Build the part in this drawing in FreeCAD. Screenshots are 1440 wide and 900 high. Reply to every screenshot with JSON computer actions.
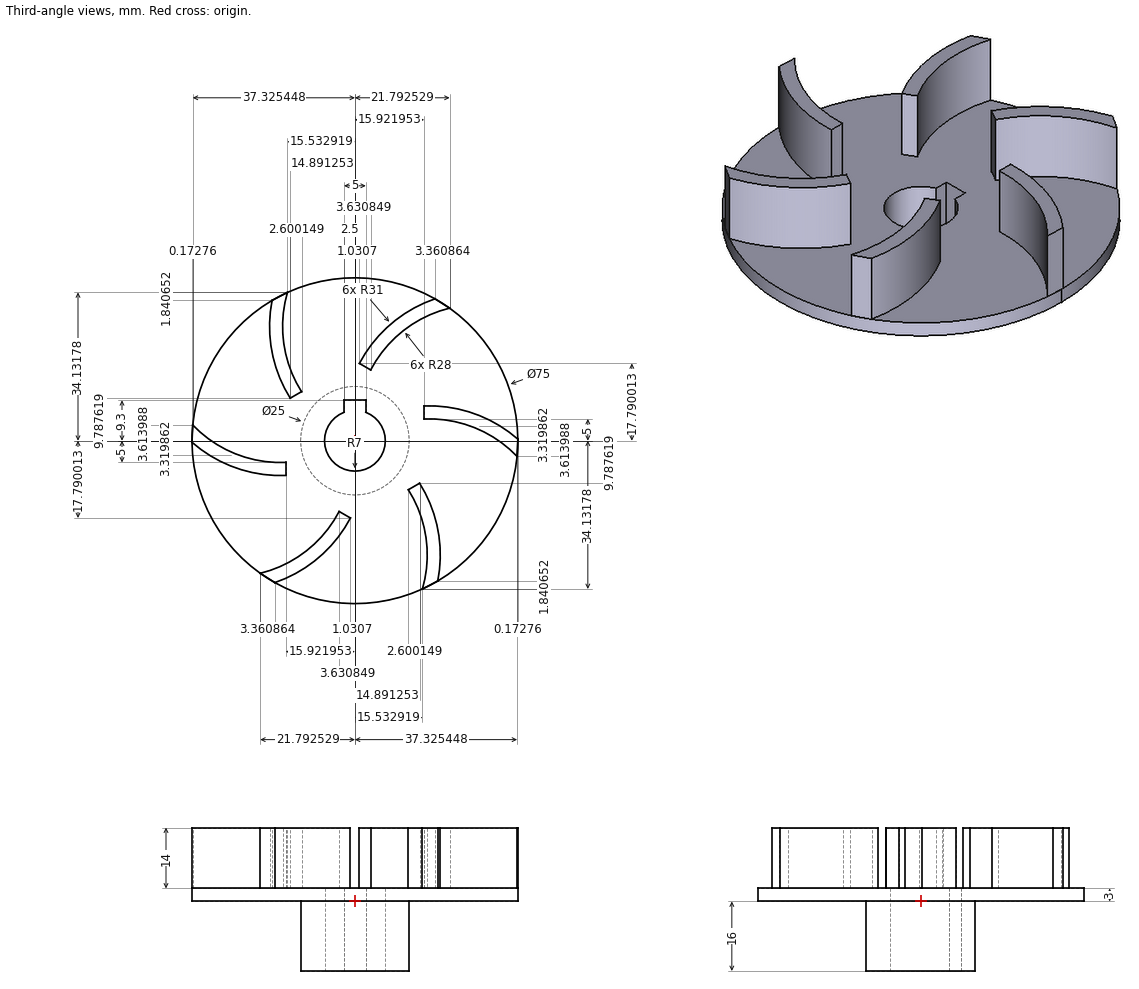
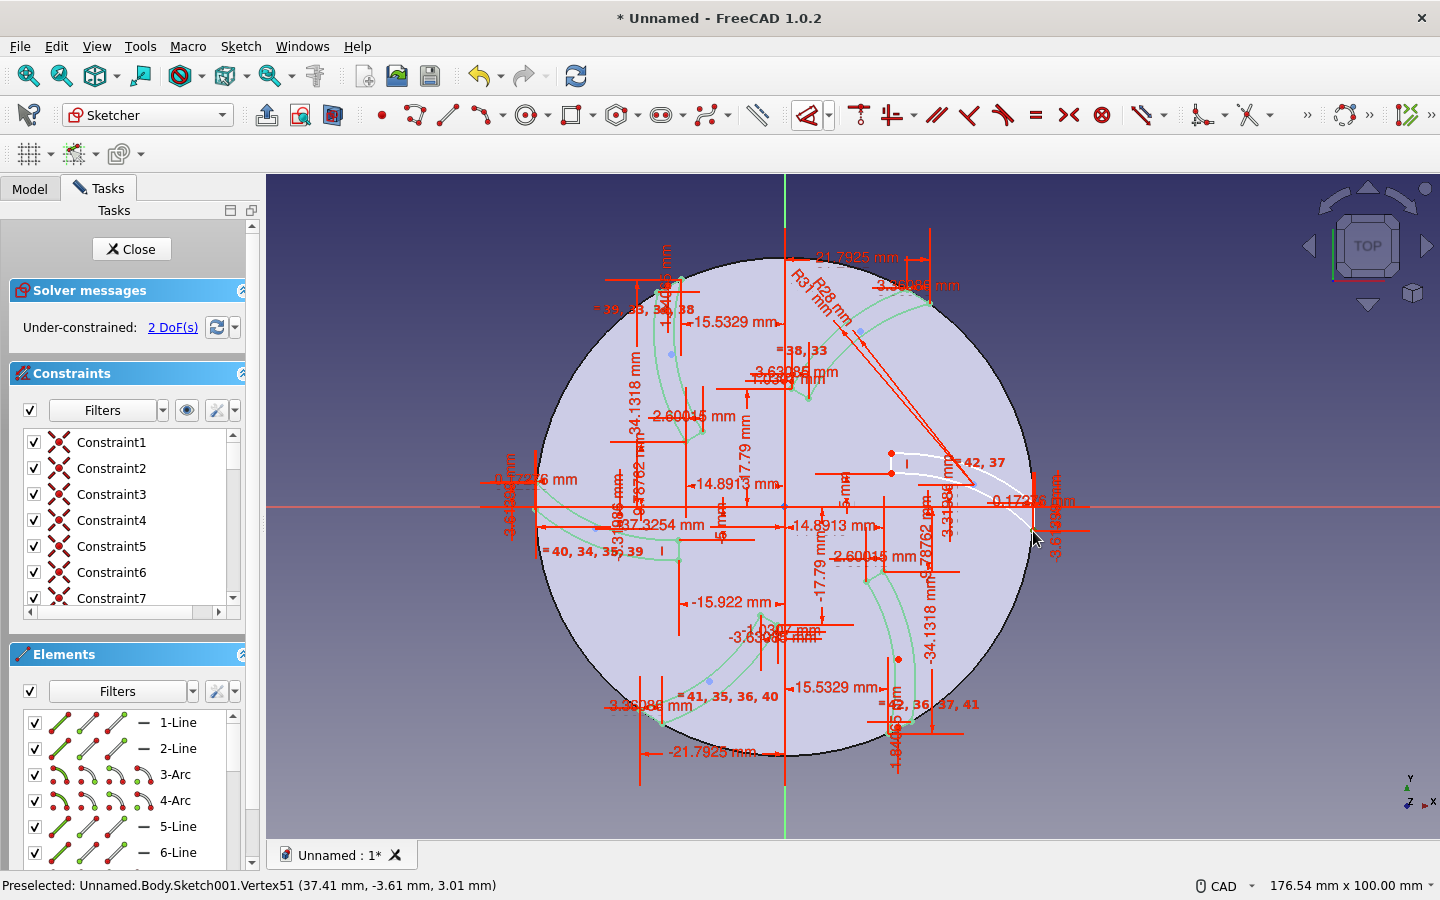
{"action": "key", "text": "l"}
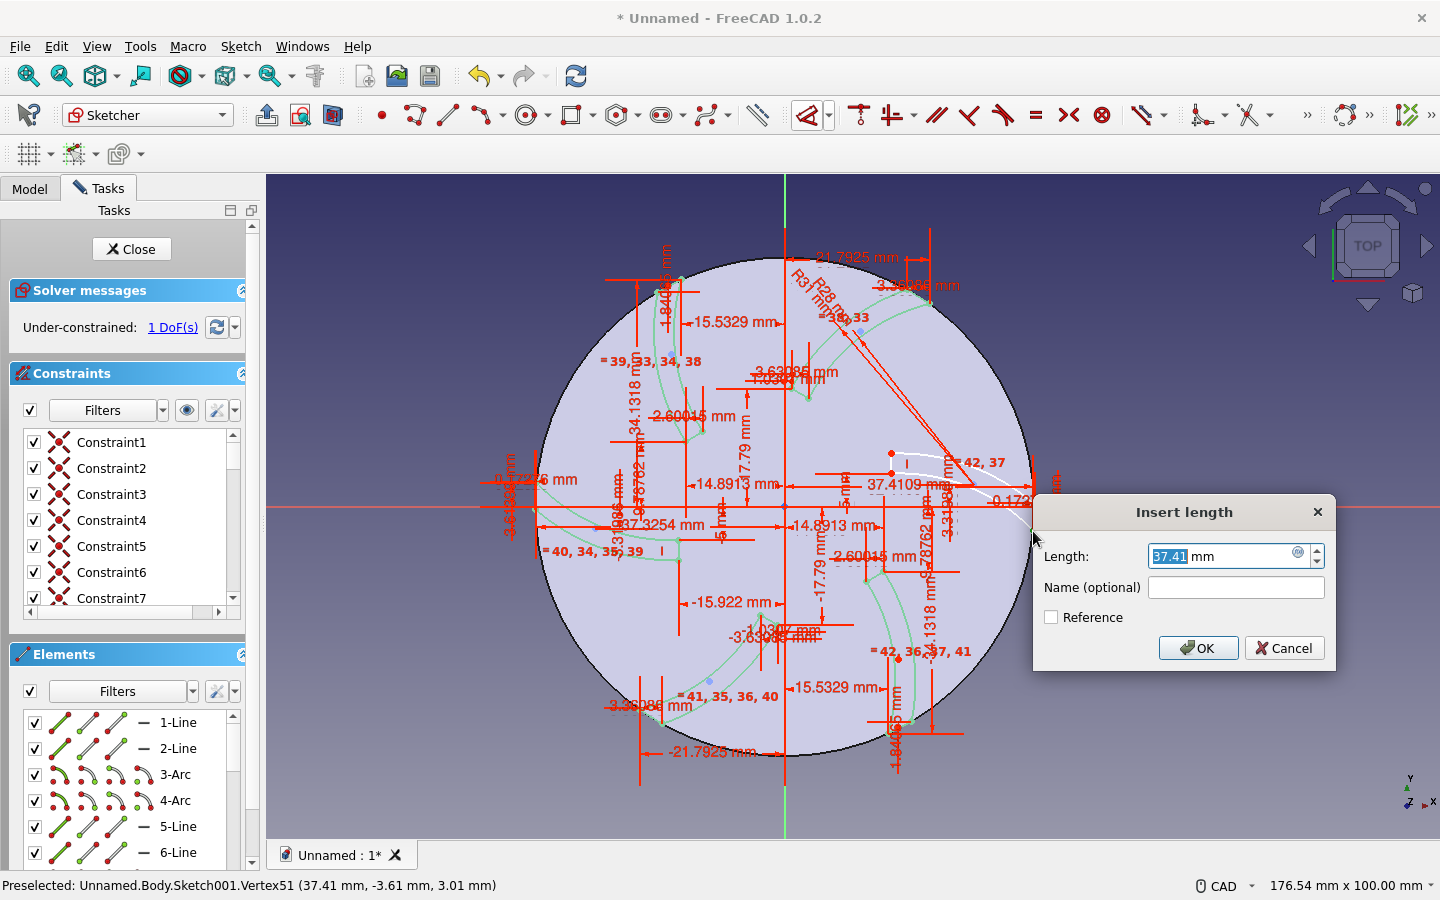
{"action": "type", "text": "37.325448"}
{"action": "key", "text": "Return"}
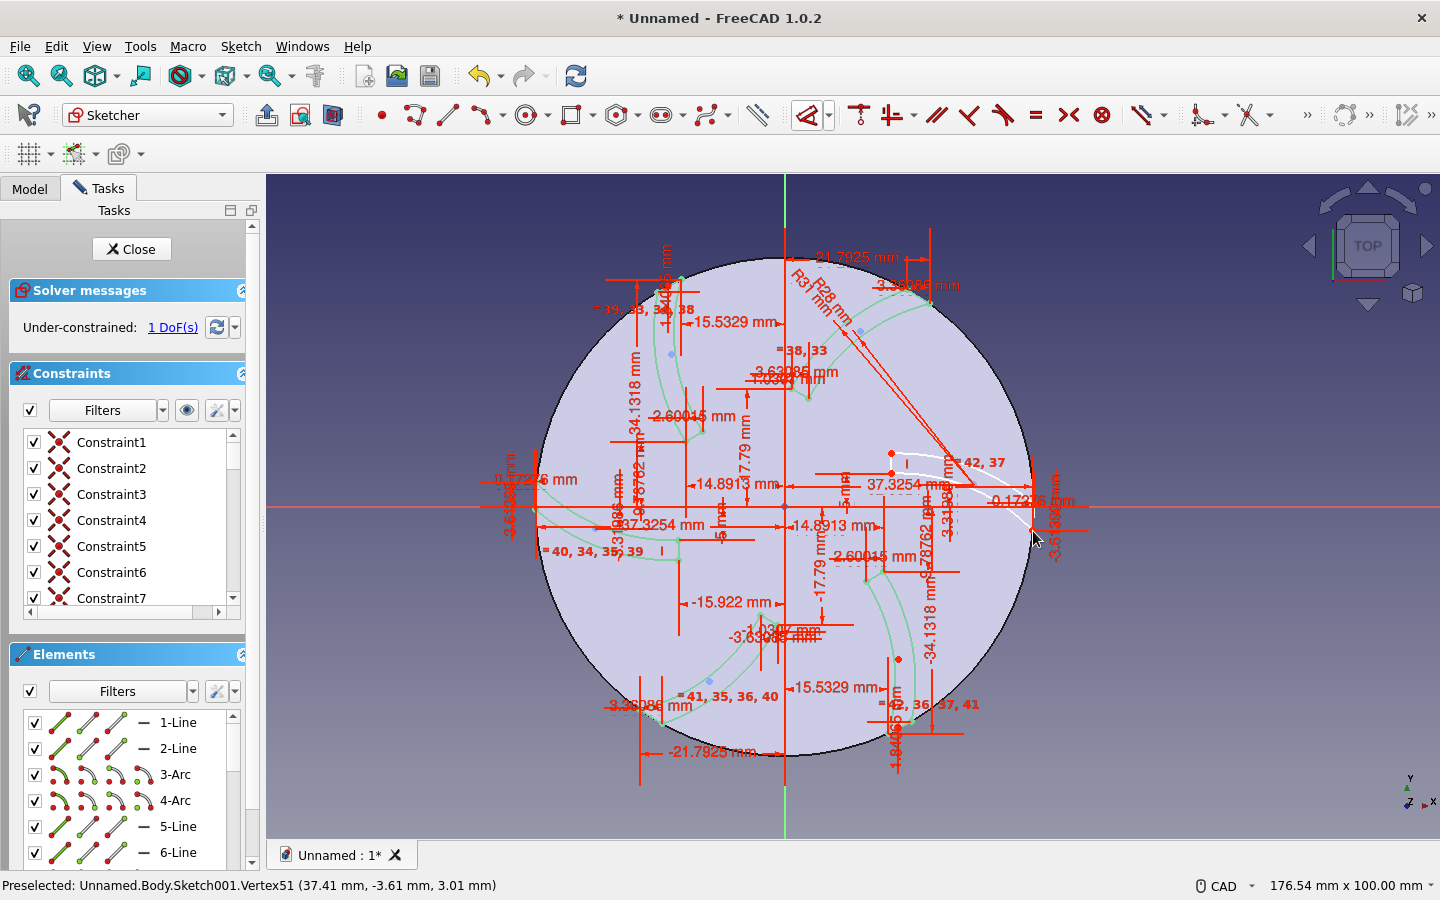
{"action": "left_click", "coordinate": [891, 454]}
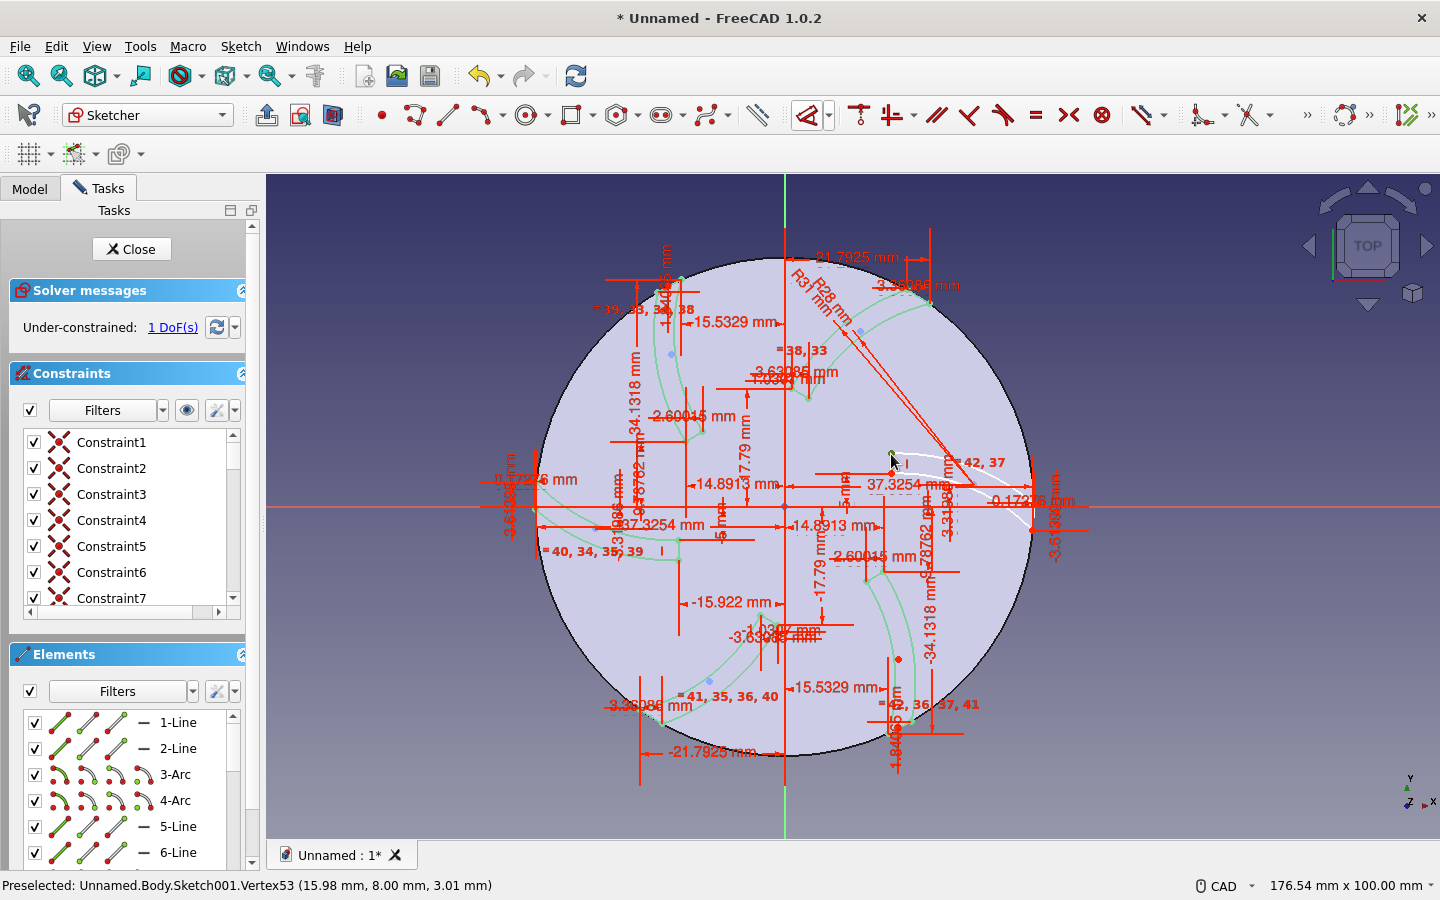
{"action": "left_click", "coordinate": [828, 116]}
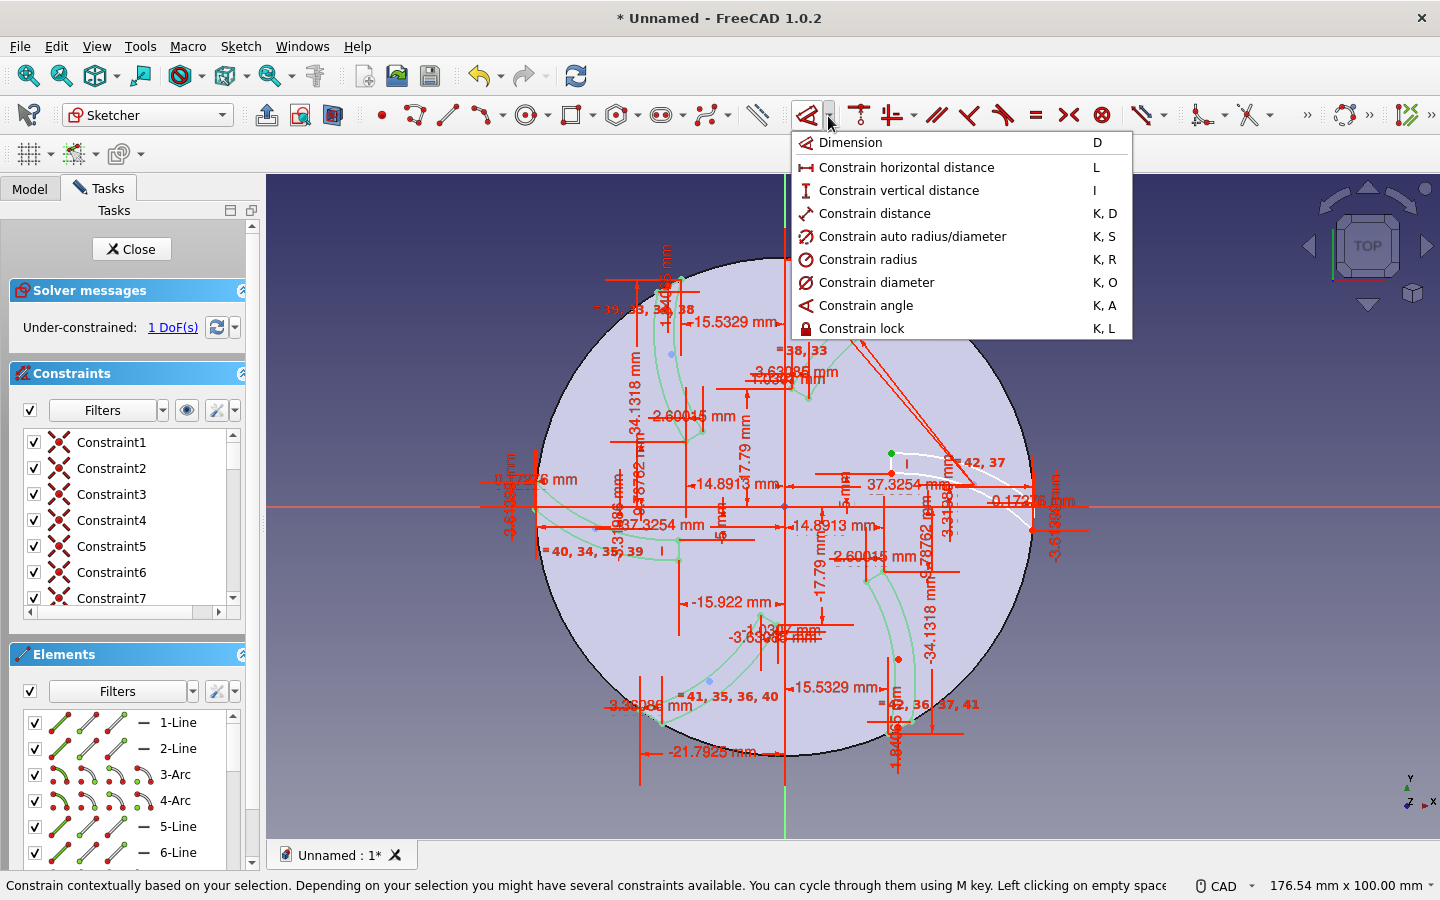
{"action": "left_click", "coordinate": [962, 168]}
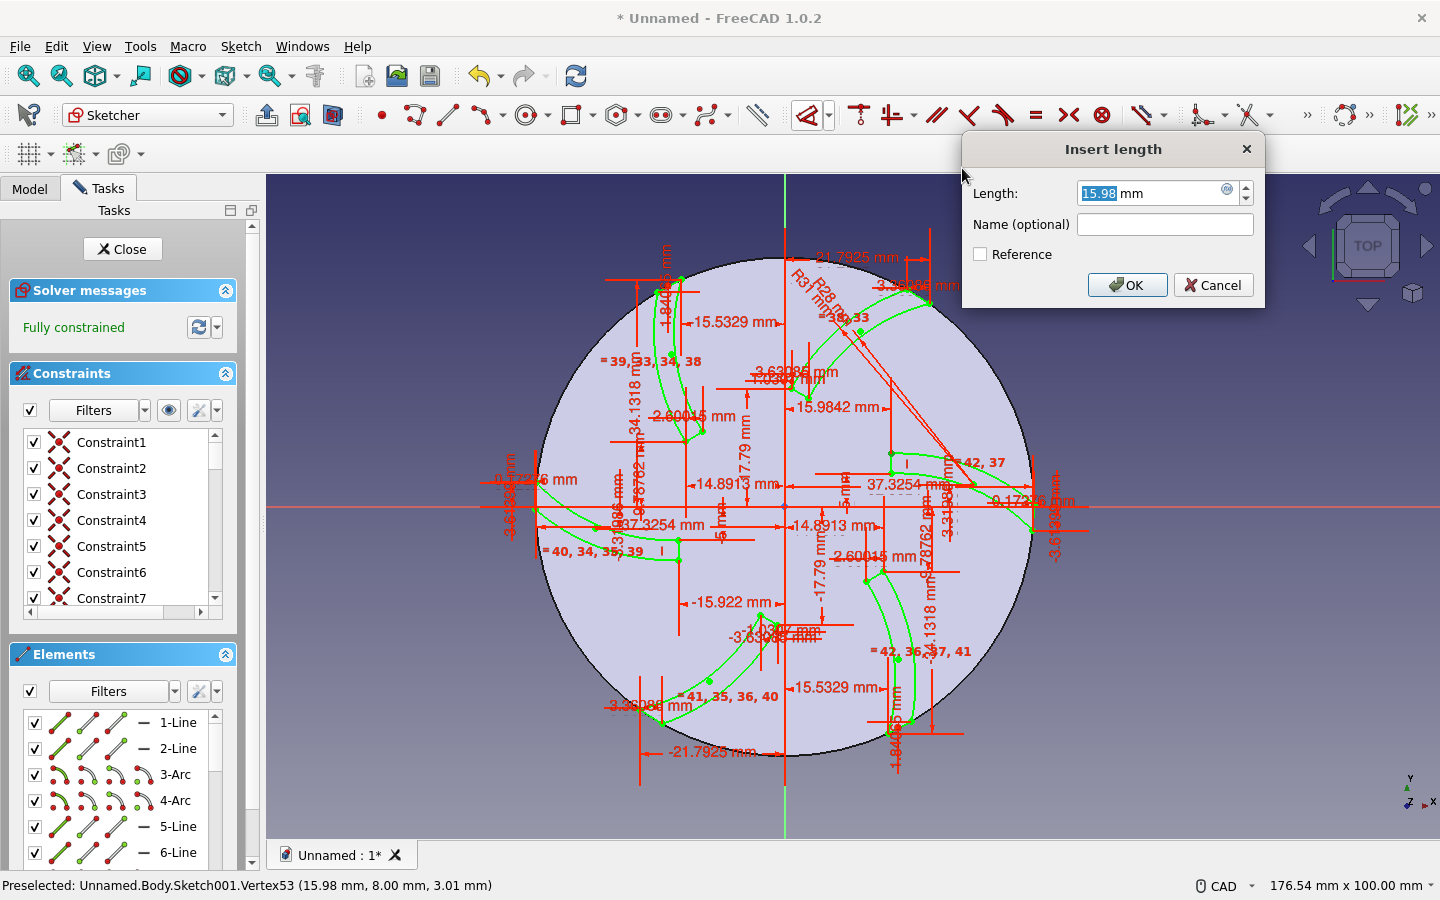
{"action": "type", "text": "15.921953"}
{"action": "key", "text": "Return"}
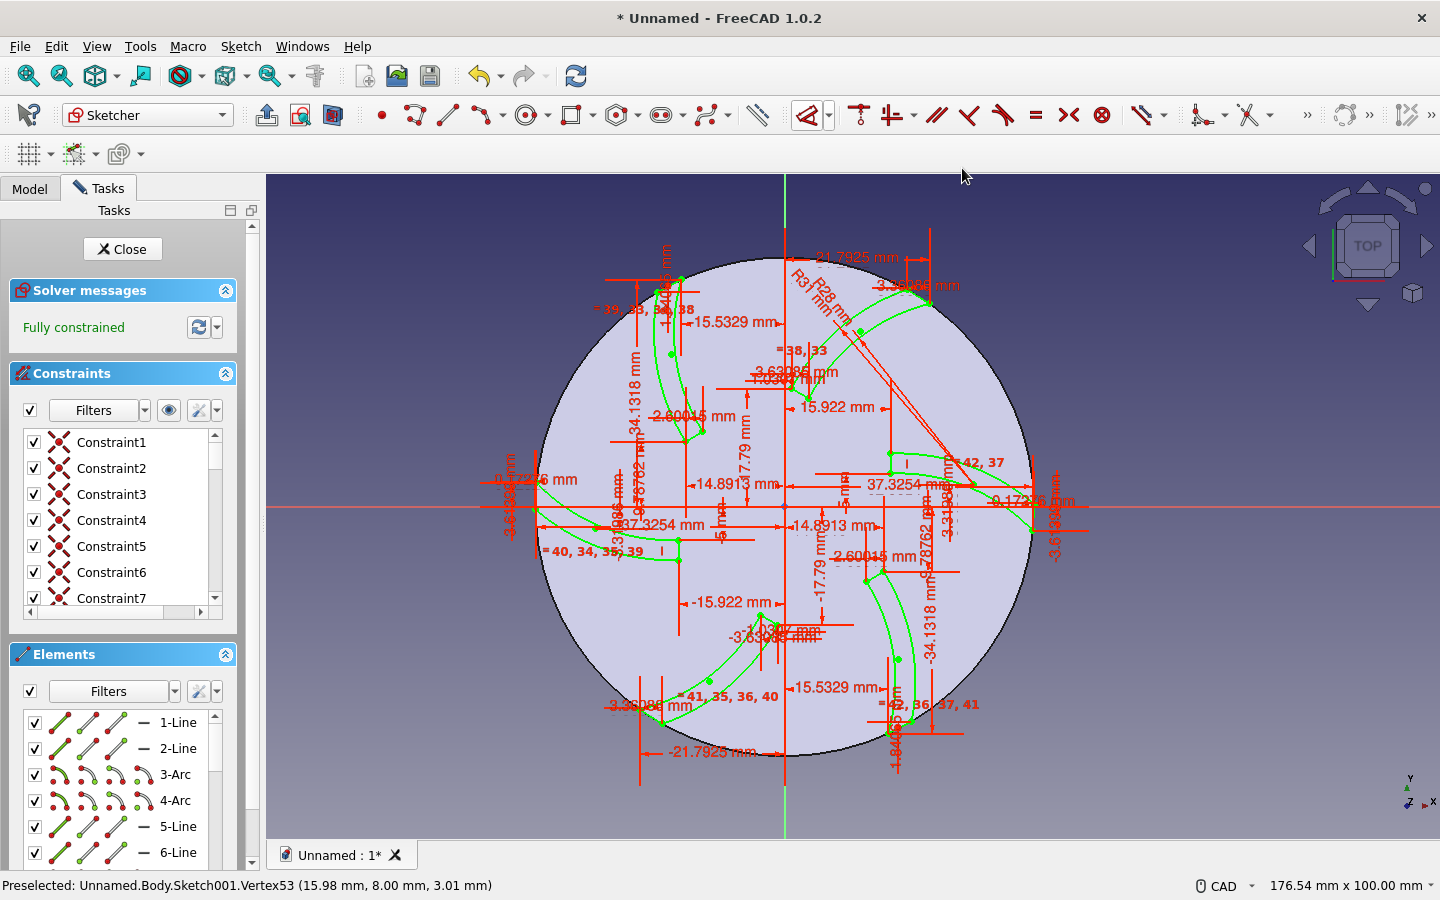
{"action": "left_click", "coordinate": [123, 249]}